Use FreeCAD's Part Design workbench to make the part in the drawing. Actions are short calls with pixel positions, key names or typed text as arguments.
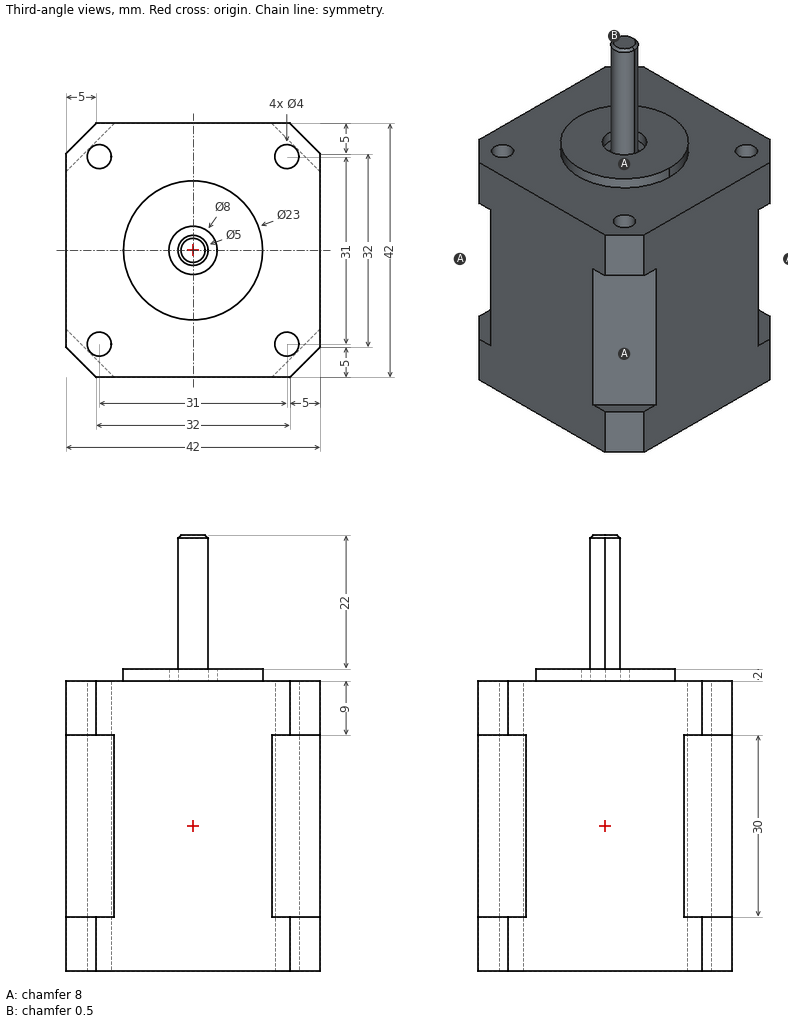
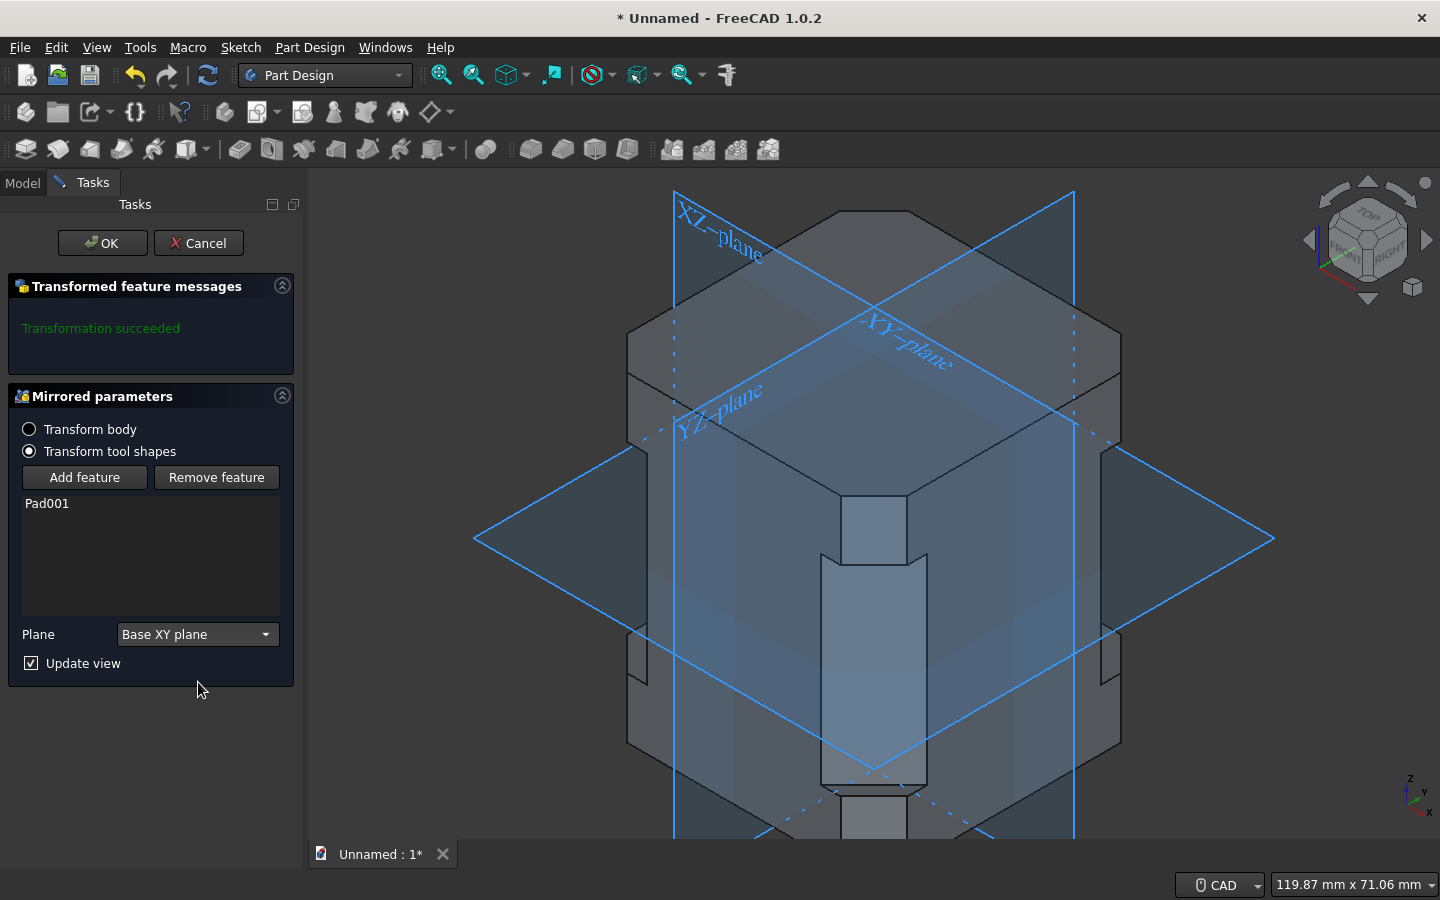
click(103, 243)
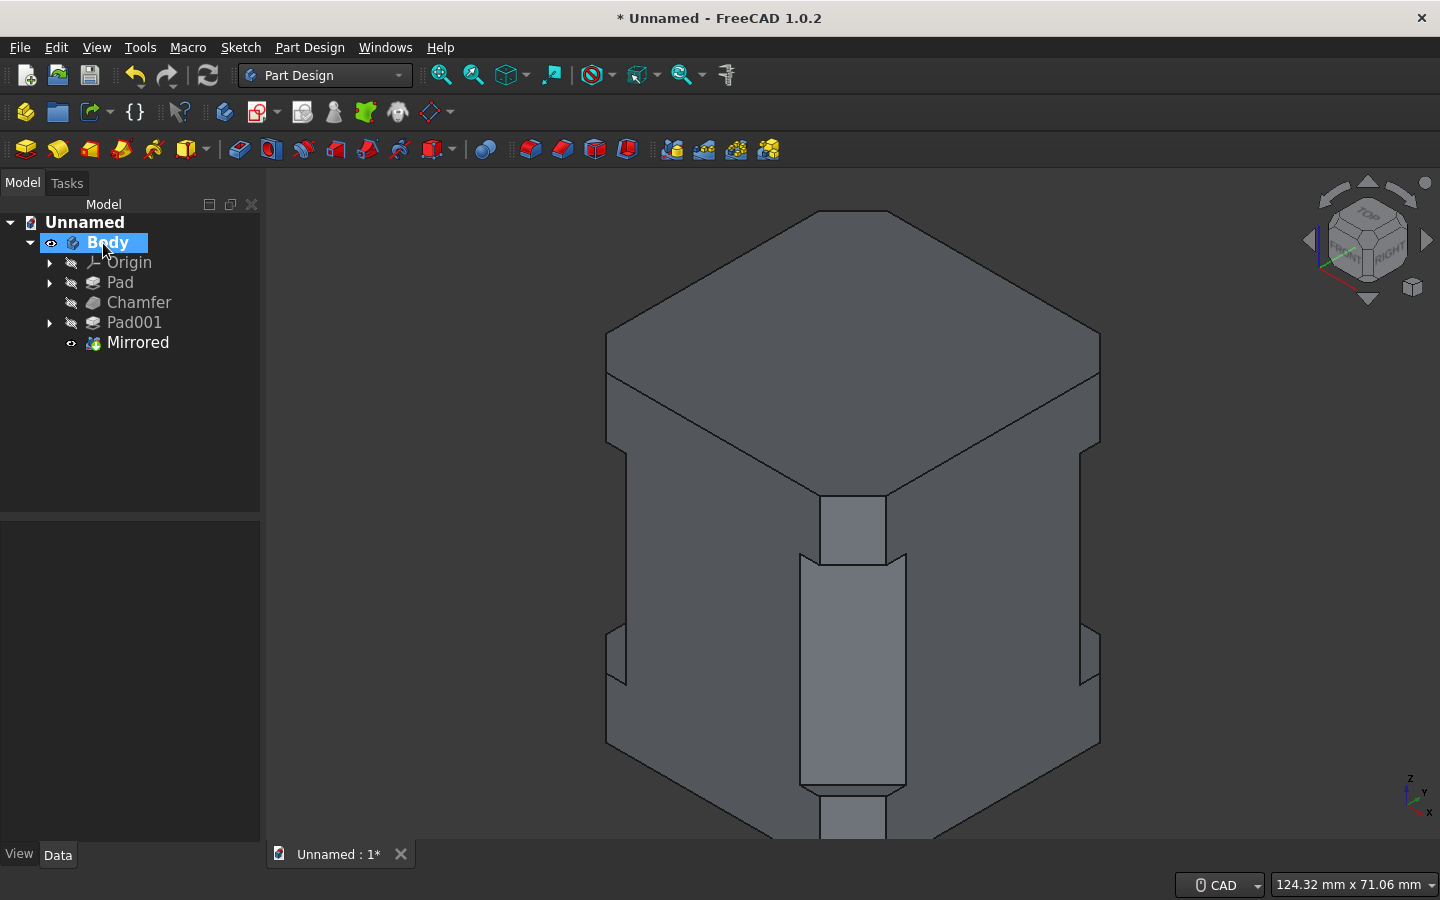
click(442, 76)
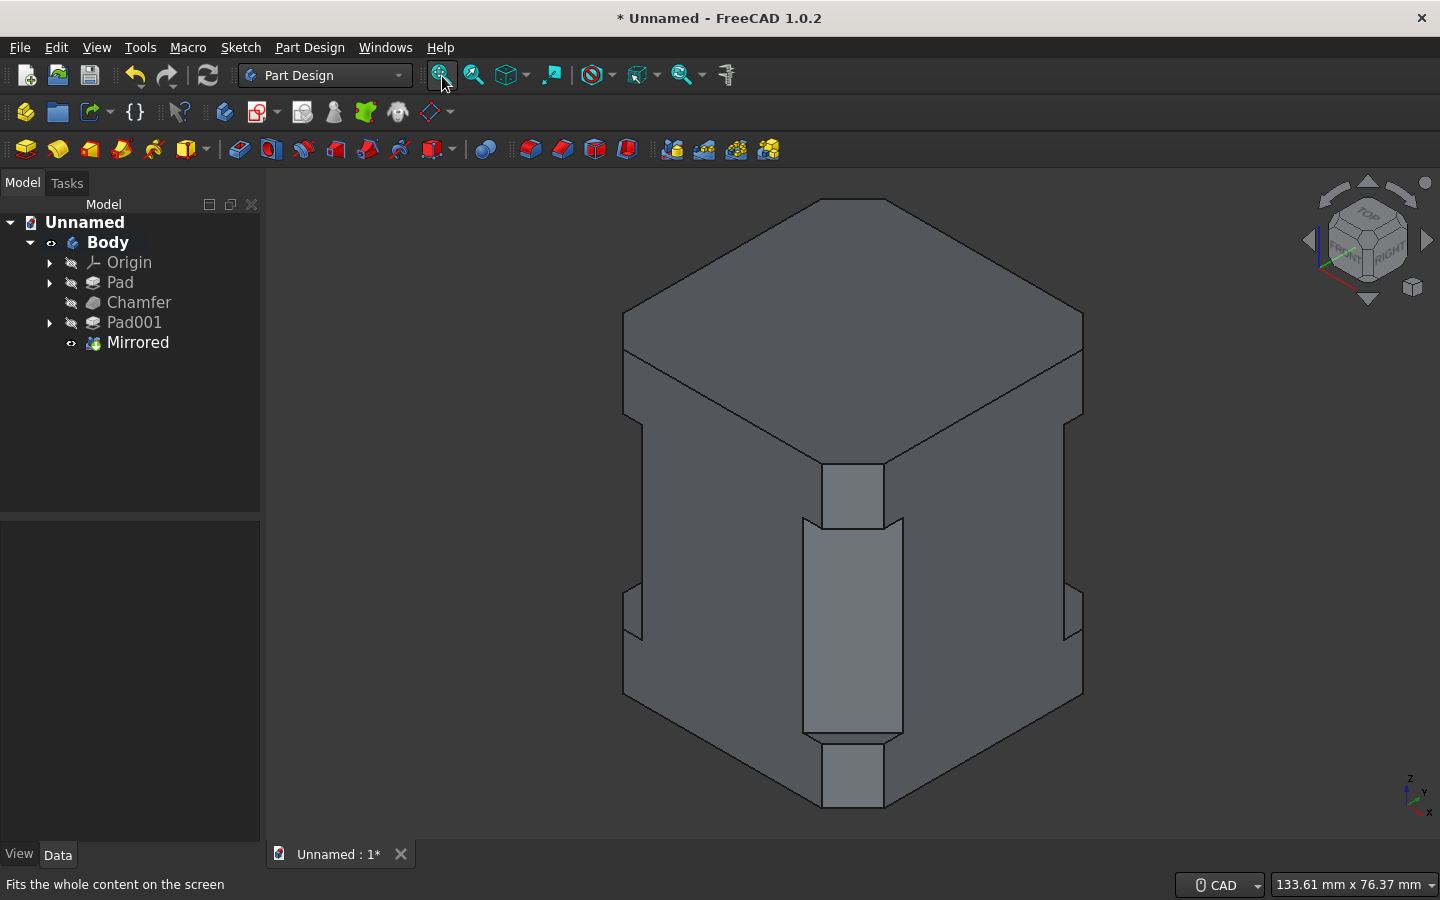
click(853, 330)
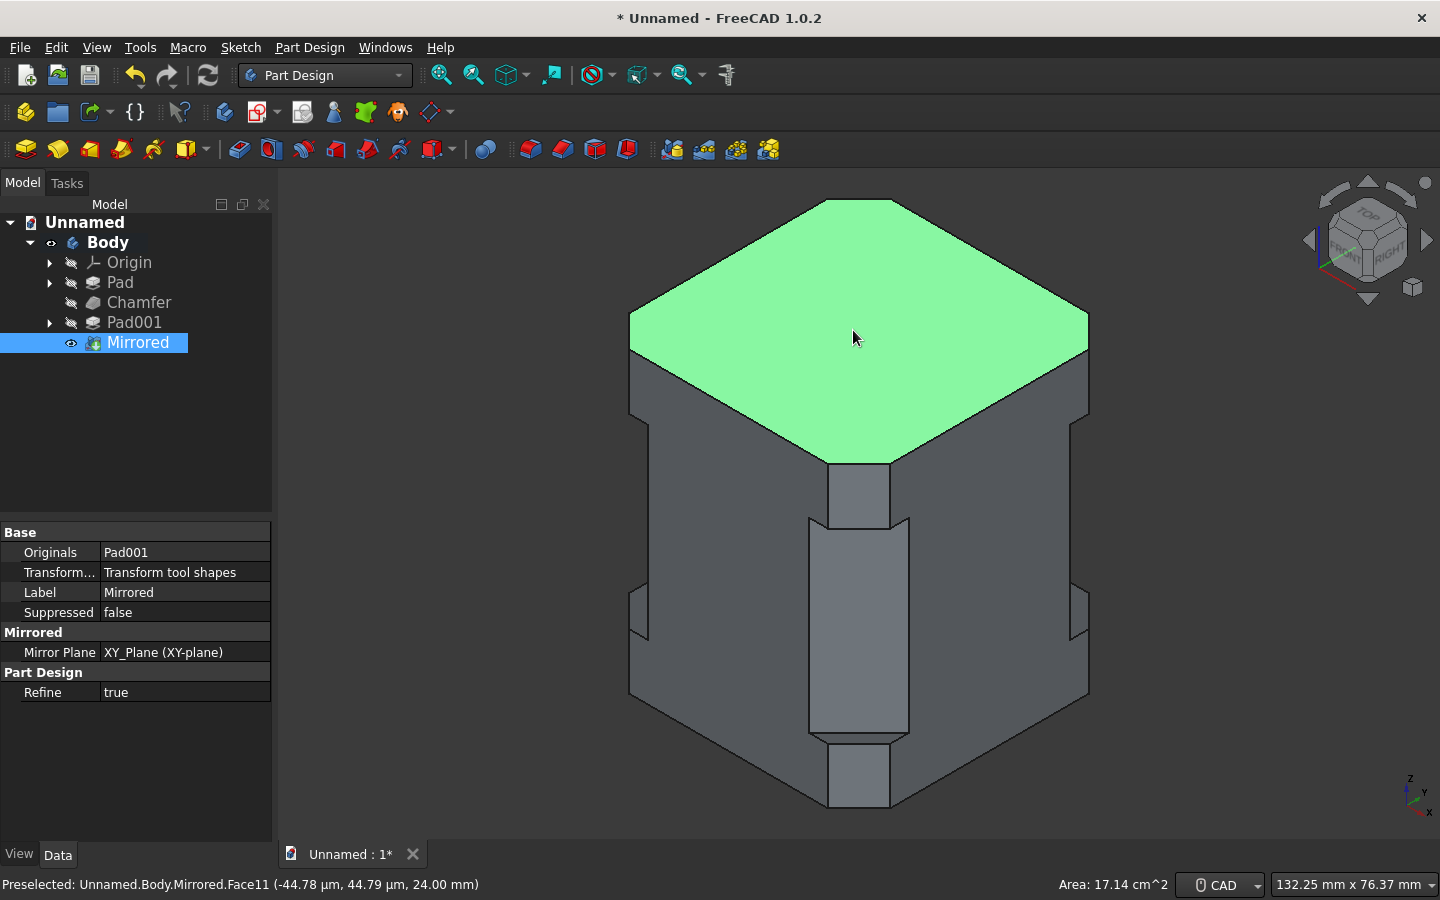
click(258, 112)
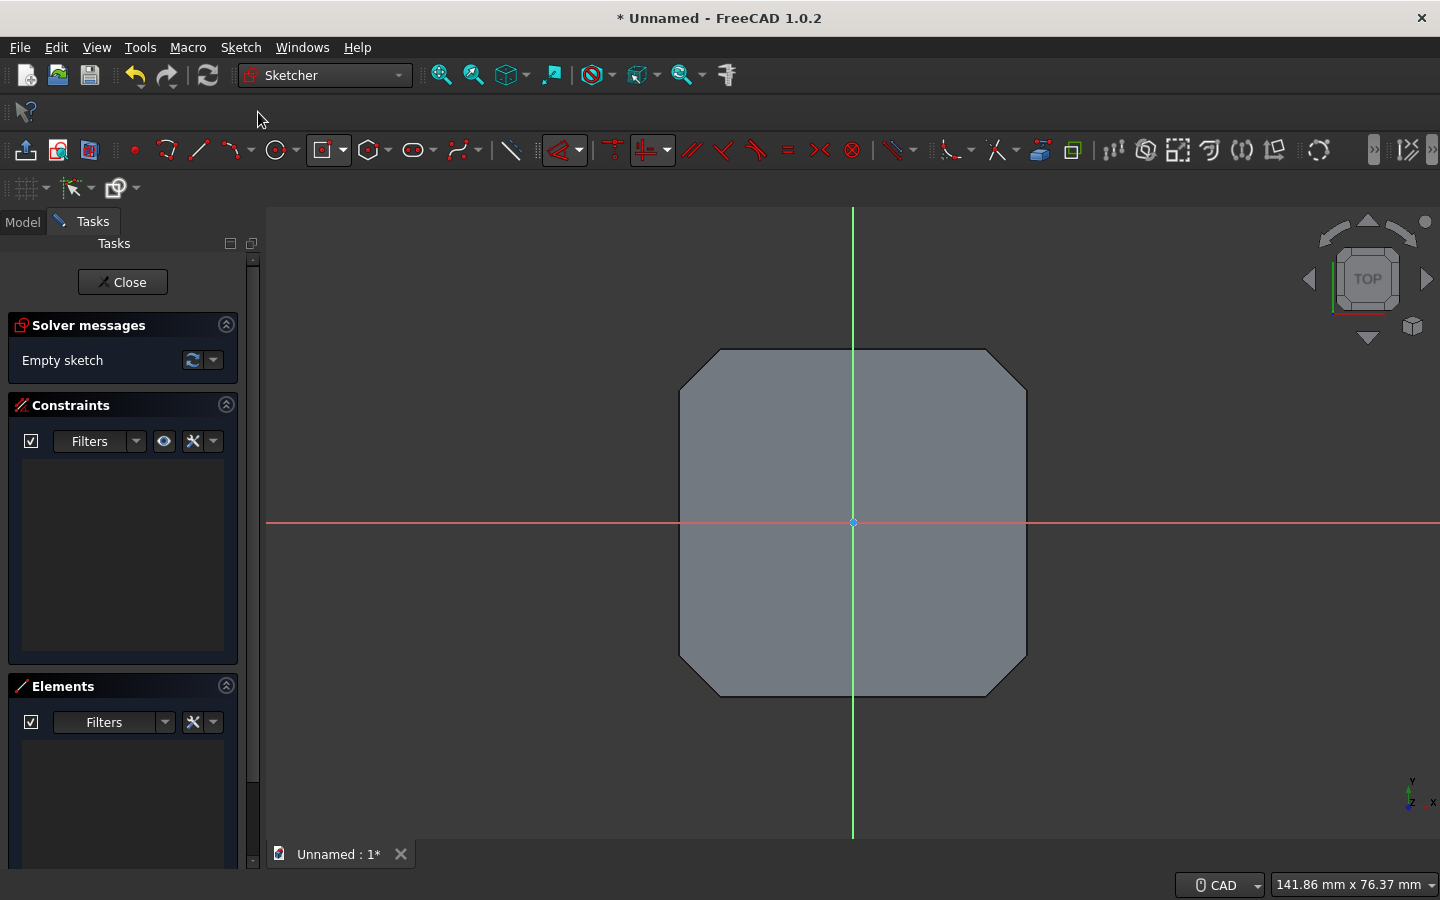
scroll(909, 523, up, 4)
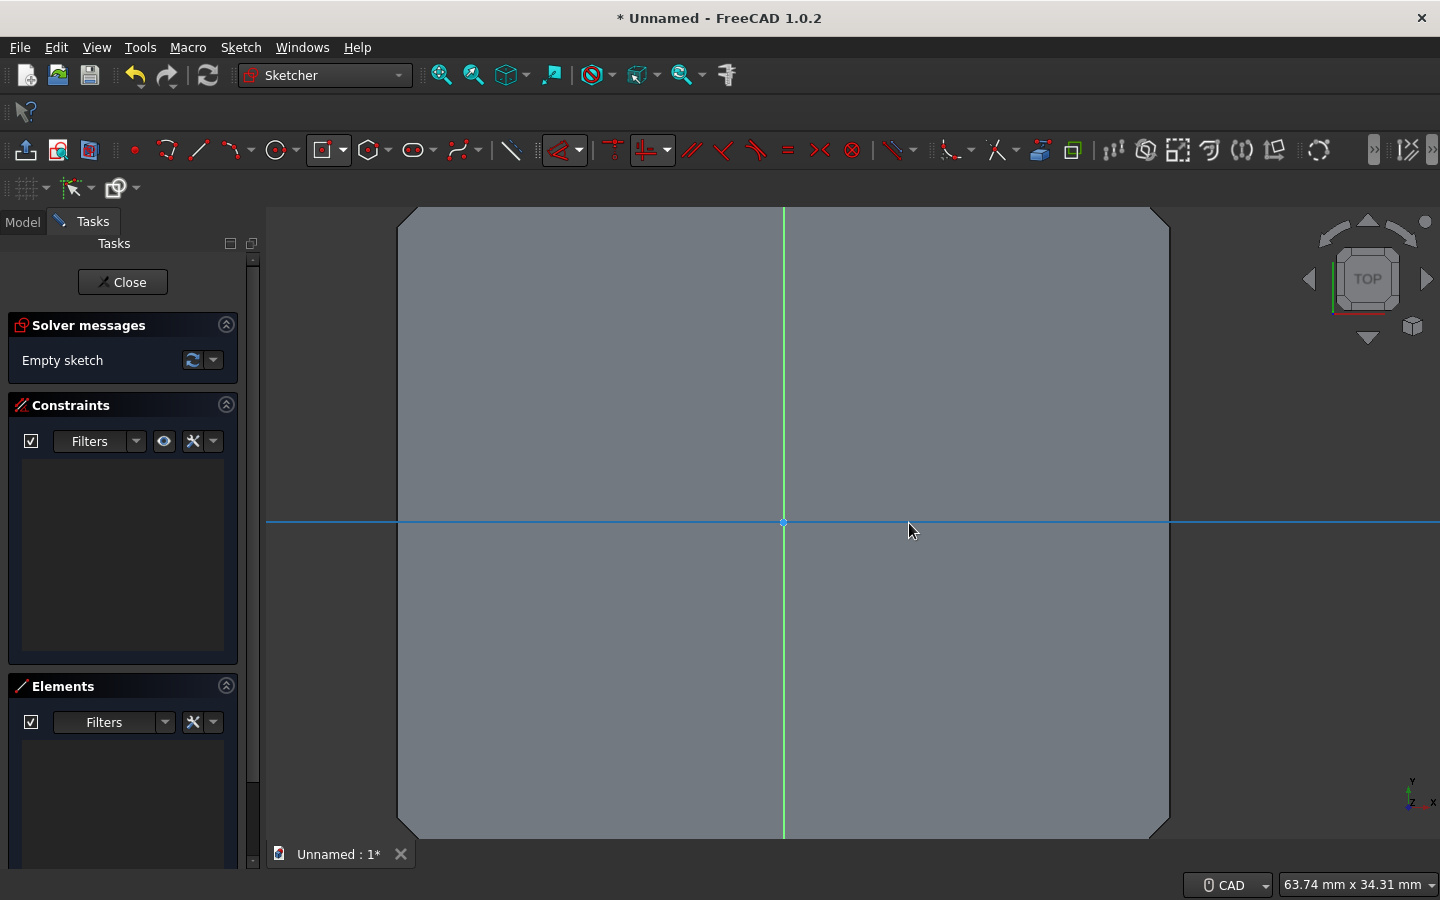
click(276, 150)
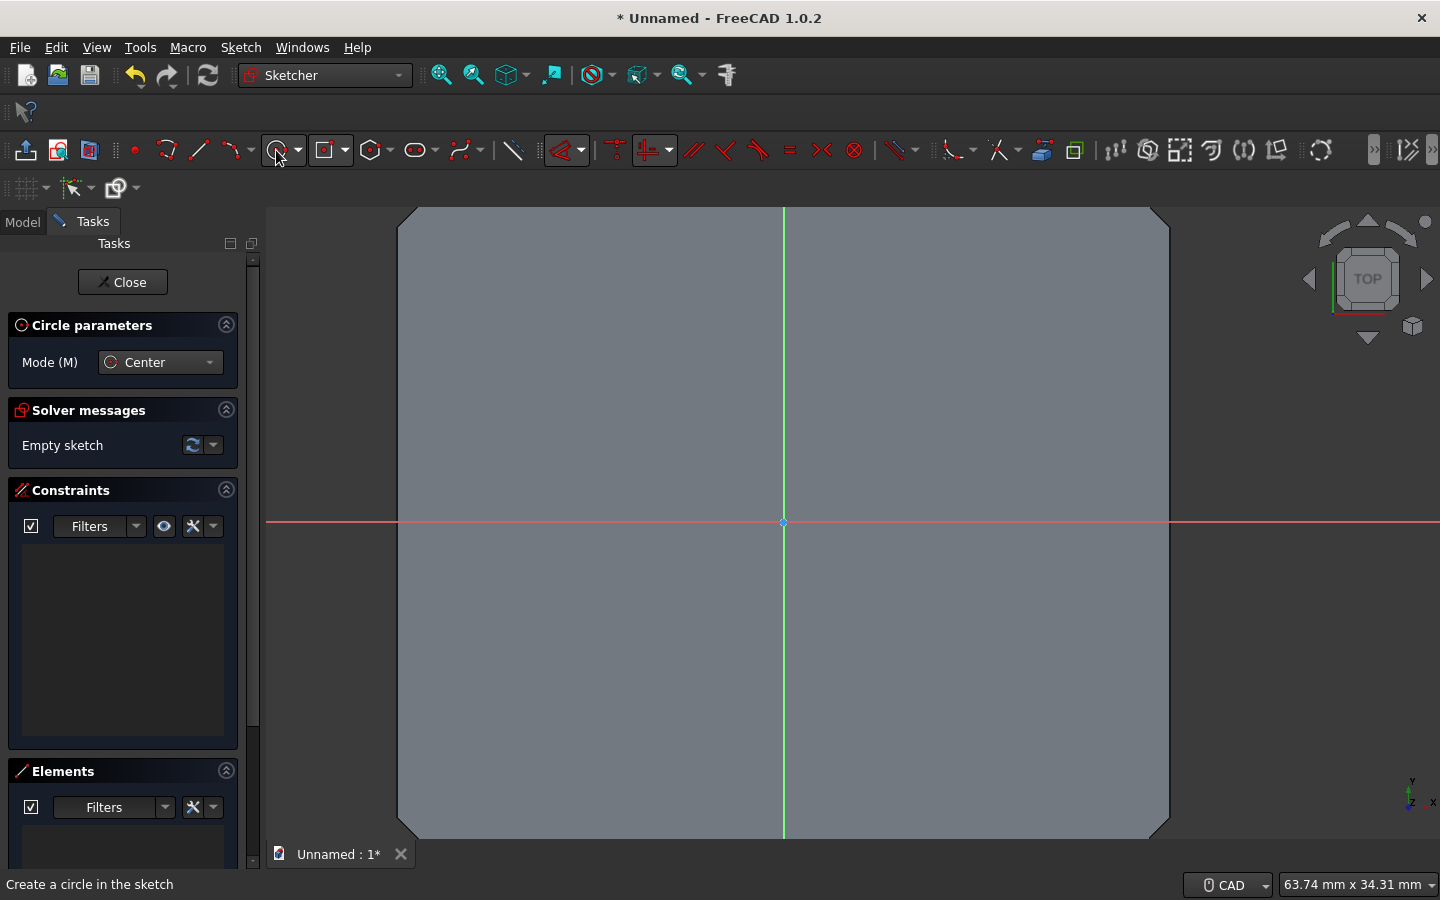
click(784, 522)
move(933, 373)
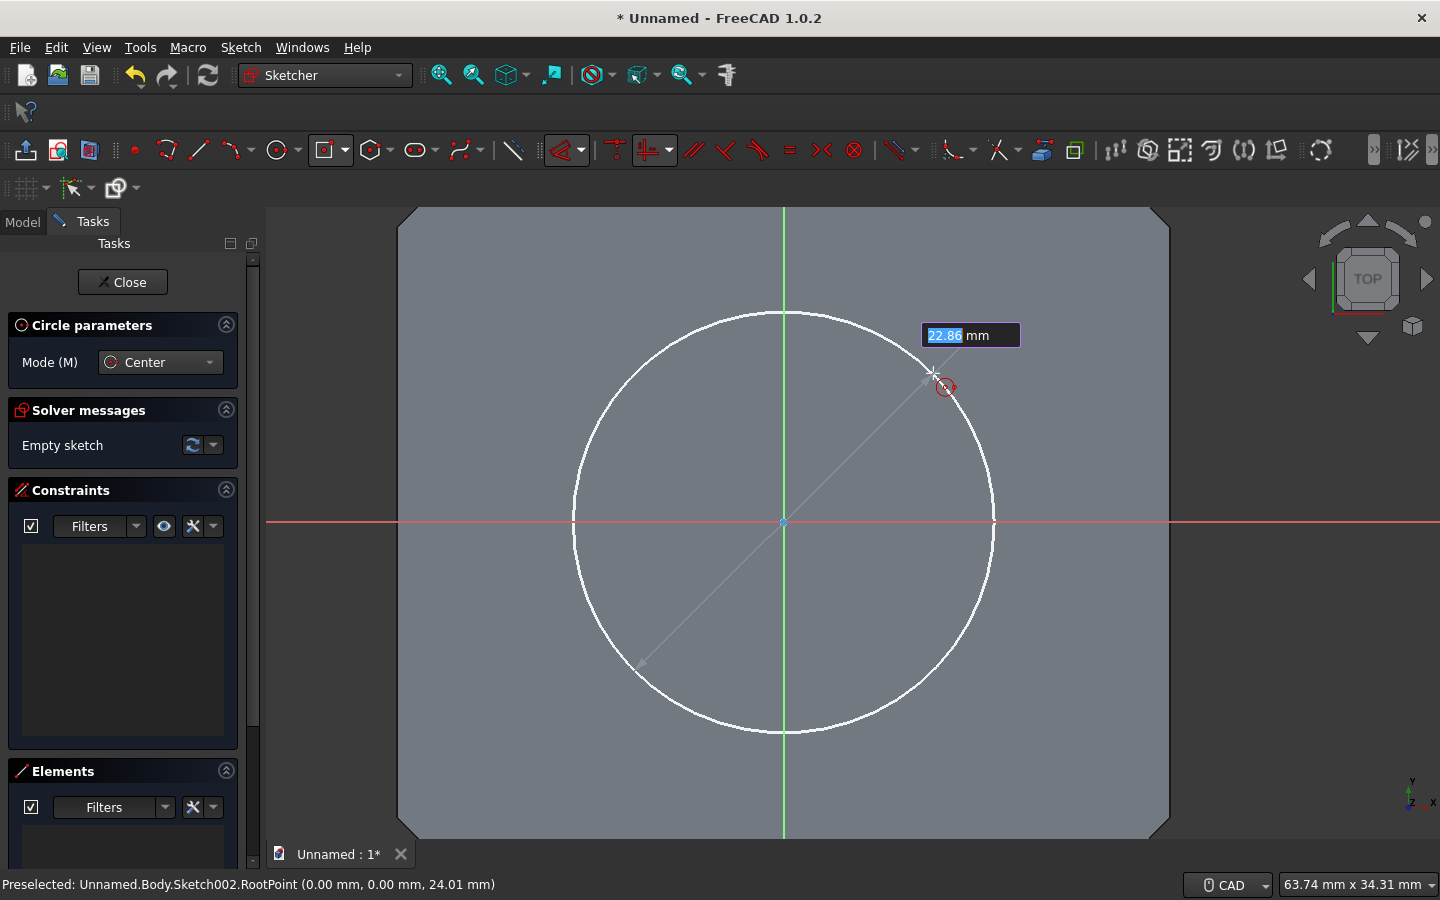
text(23)
key(Return)
key(Escape)